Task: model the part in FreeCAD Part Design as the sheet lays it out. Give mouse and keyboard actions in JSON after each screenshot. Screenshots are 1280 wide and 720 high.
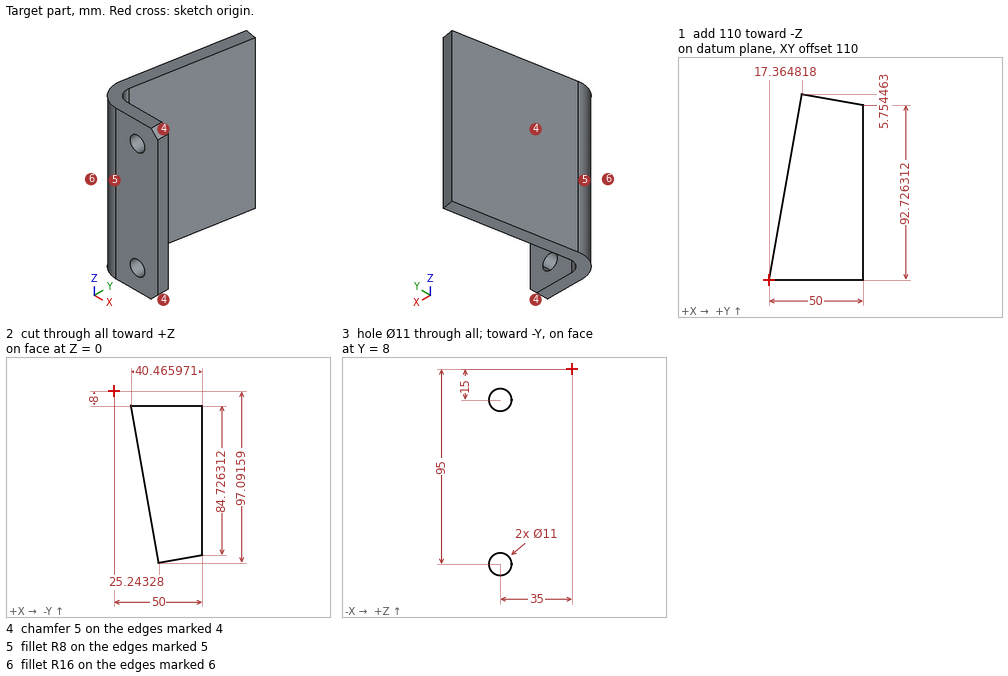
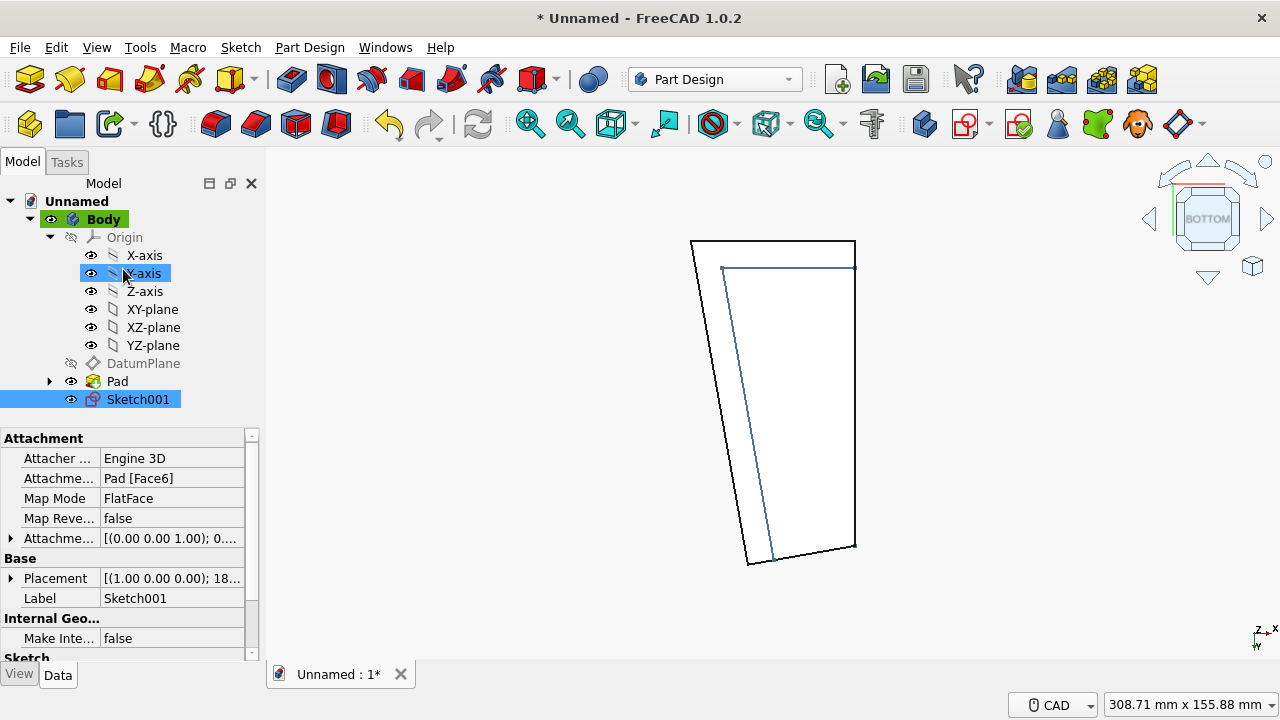
{"action": "left_click", "coordinate": [292, 80]}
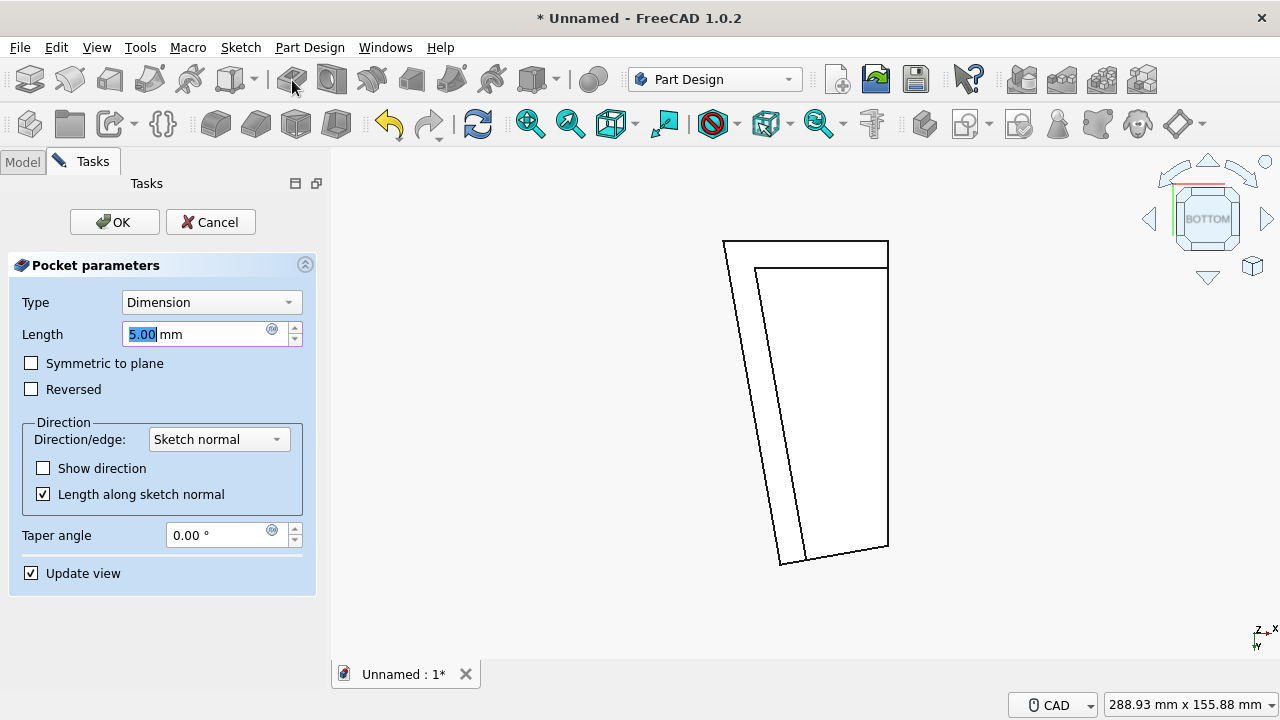
{"action": "left_click", "coordinate": [212, 302]}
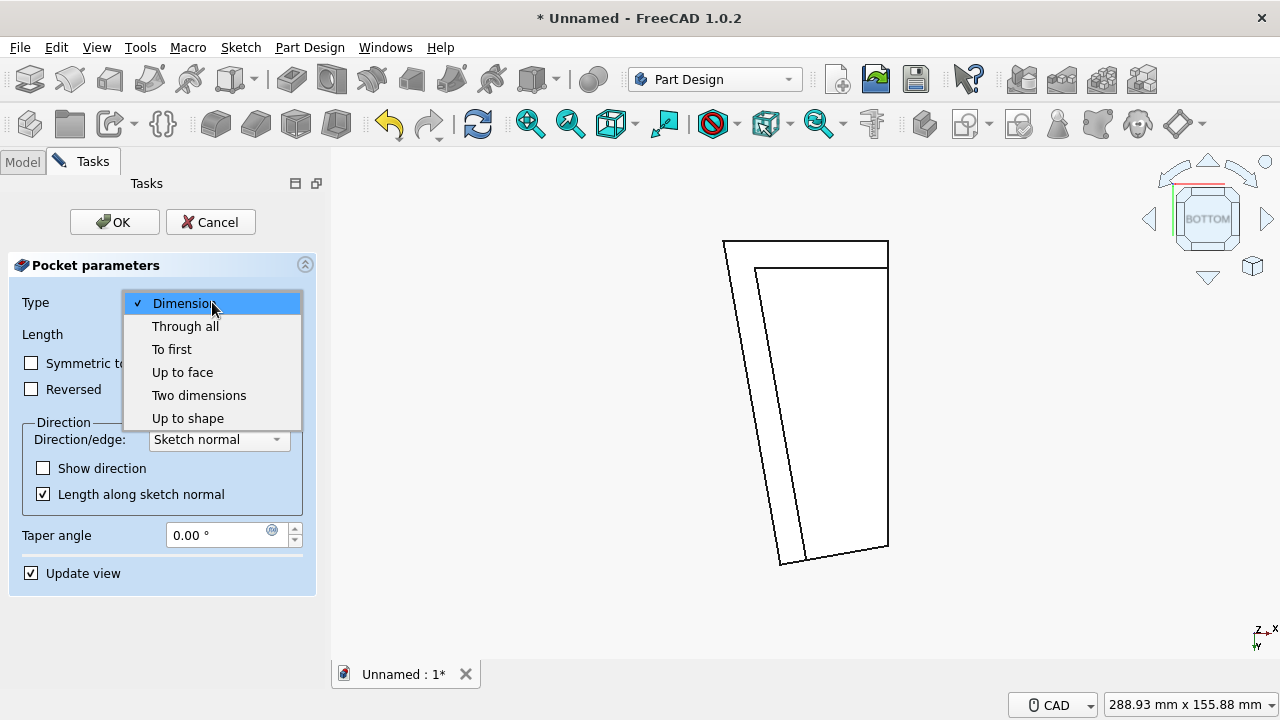
{"action": "left_click", "coordinate": [212, 326]}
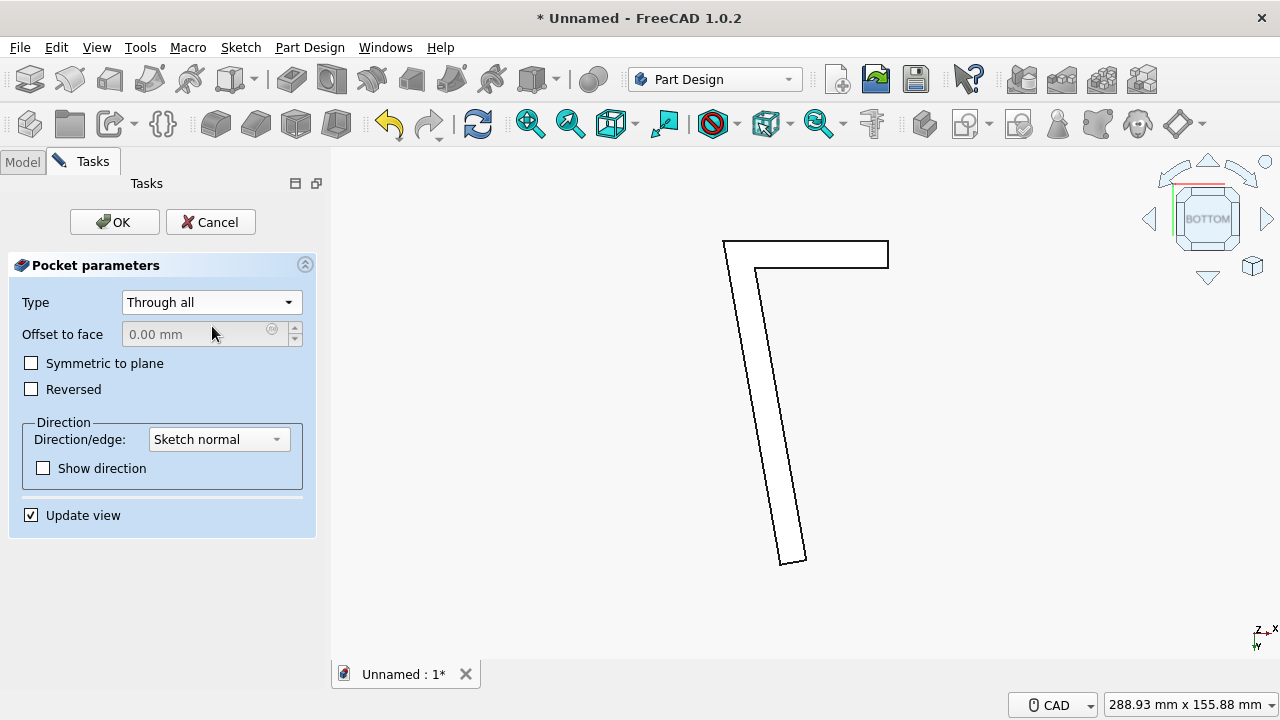
{"action": "left_click", "coordinate": [115, 222]}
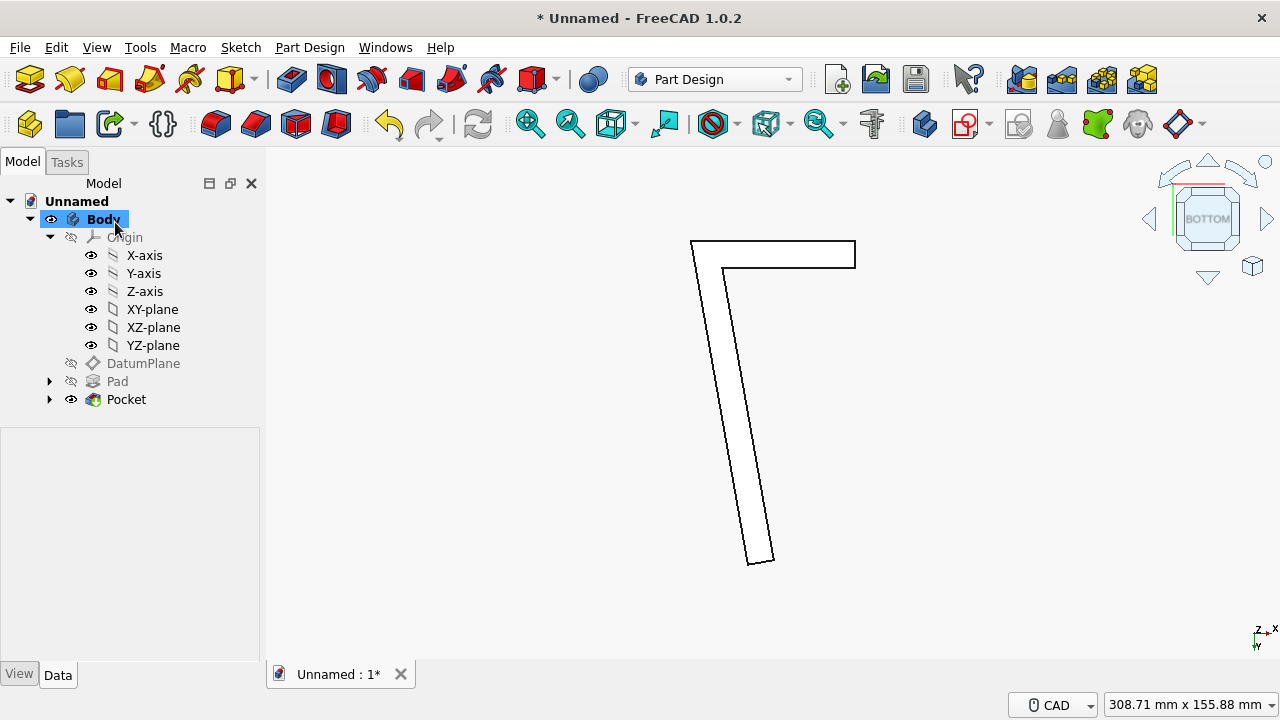
{"action": "key", "text": "4"}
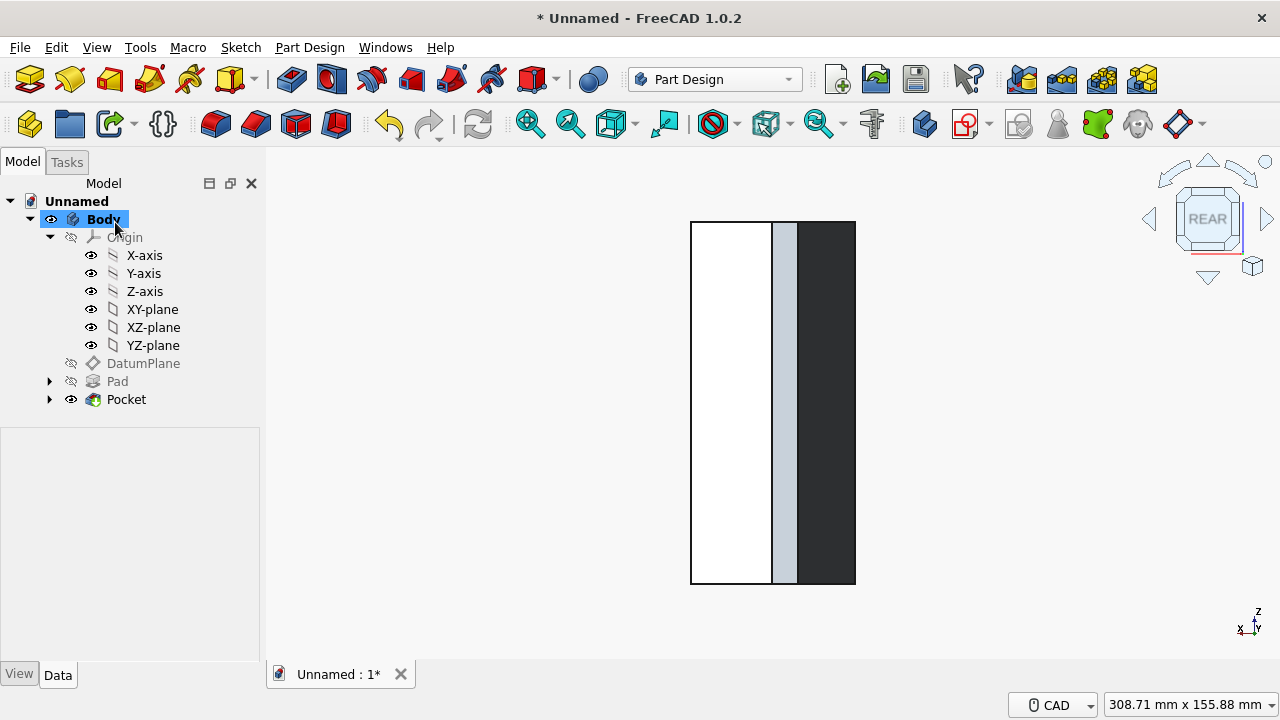
{"action": "left_click", "coordinate": [757, 299]}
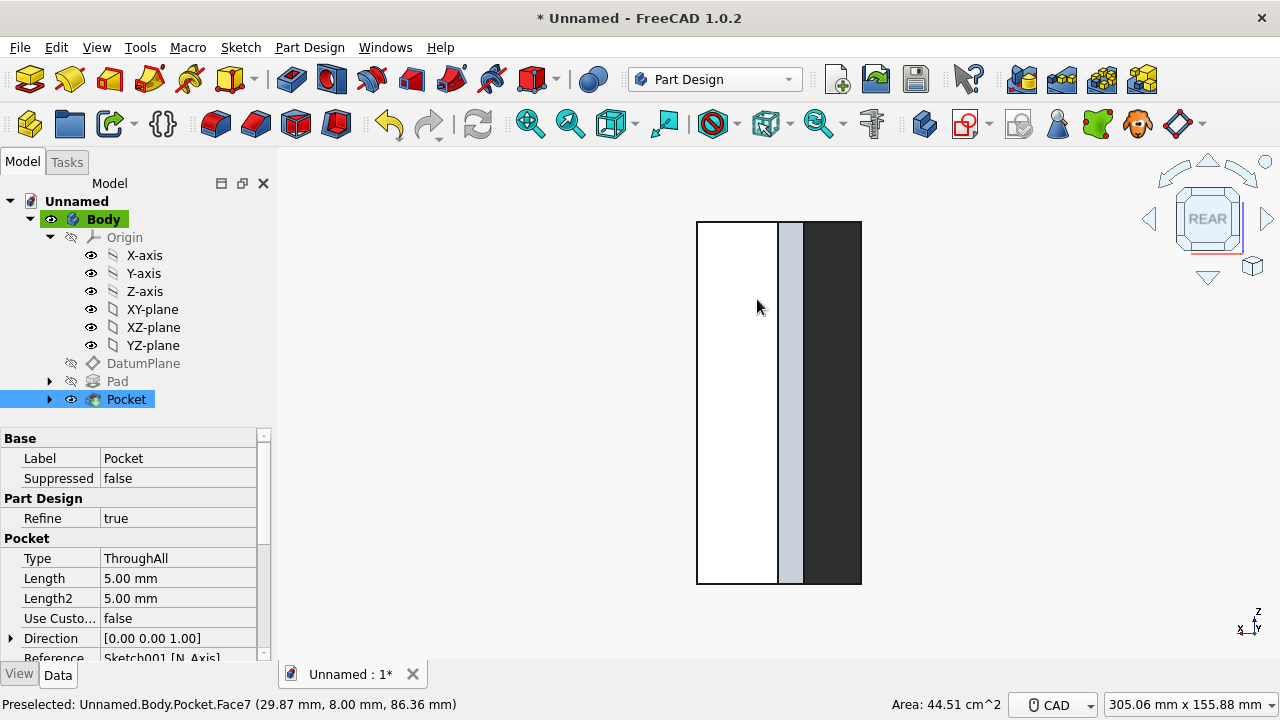
{"action": "left_click", "coordinate": [966, 124]}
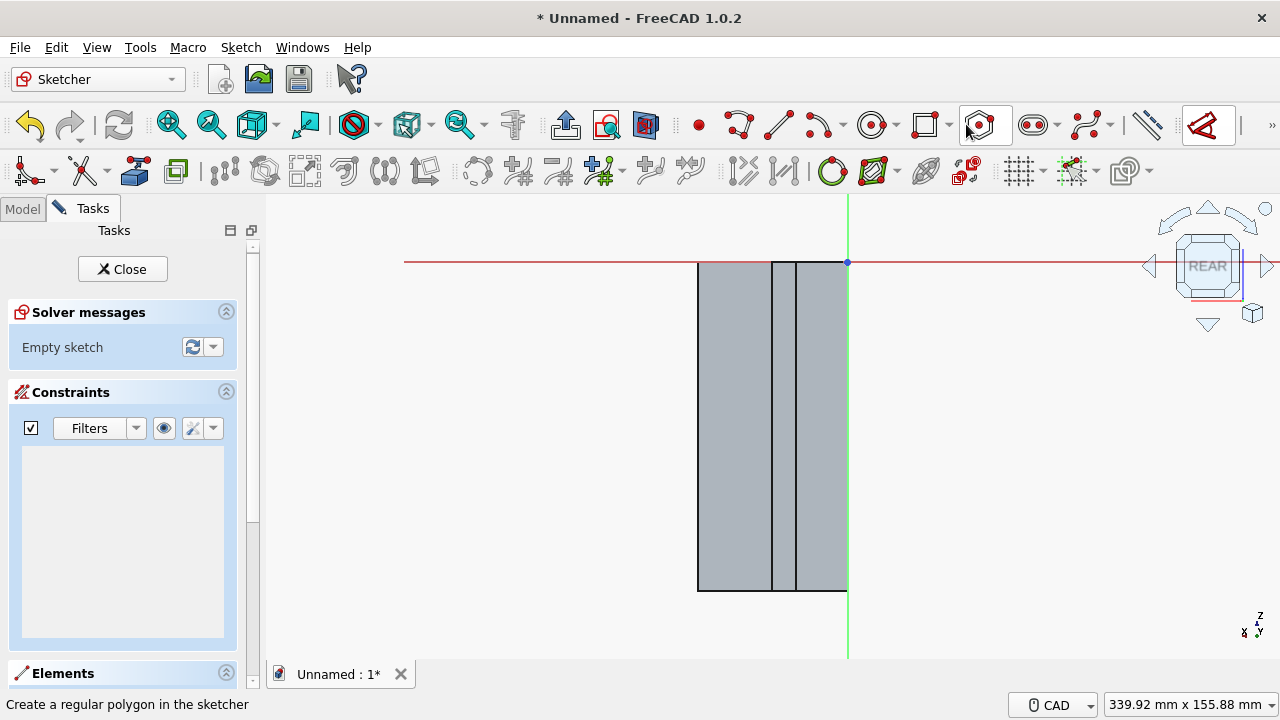
{"action": "left_click", "coordinate": [872, 126]}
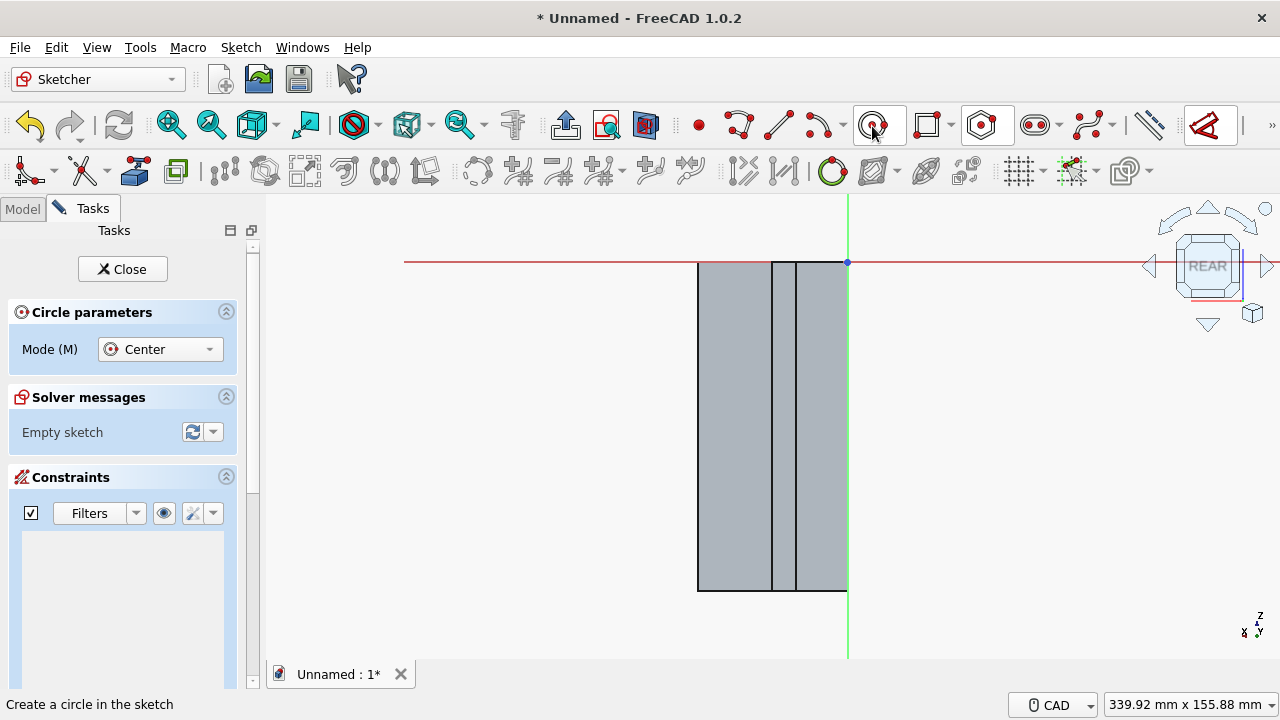
{"action": "scroll", "coordinate": [743, 546], "scroll_direction": "up", "scroll_amount": 2}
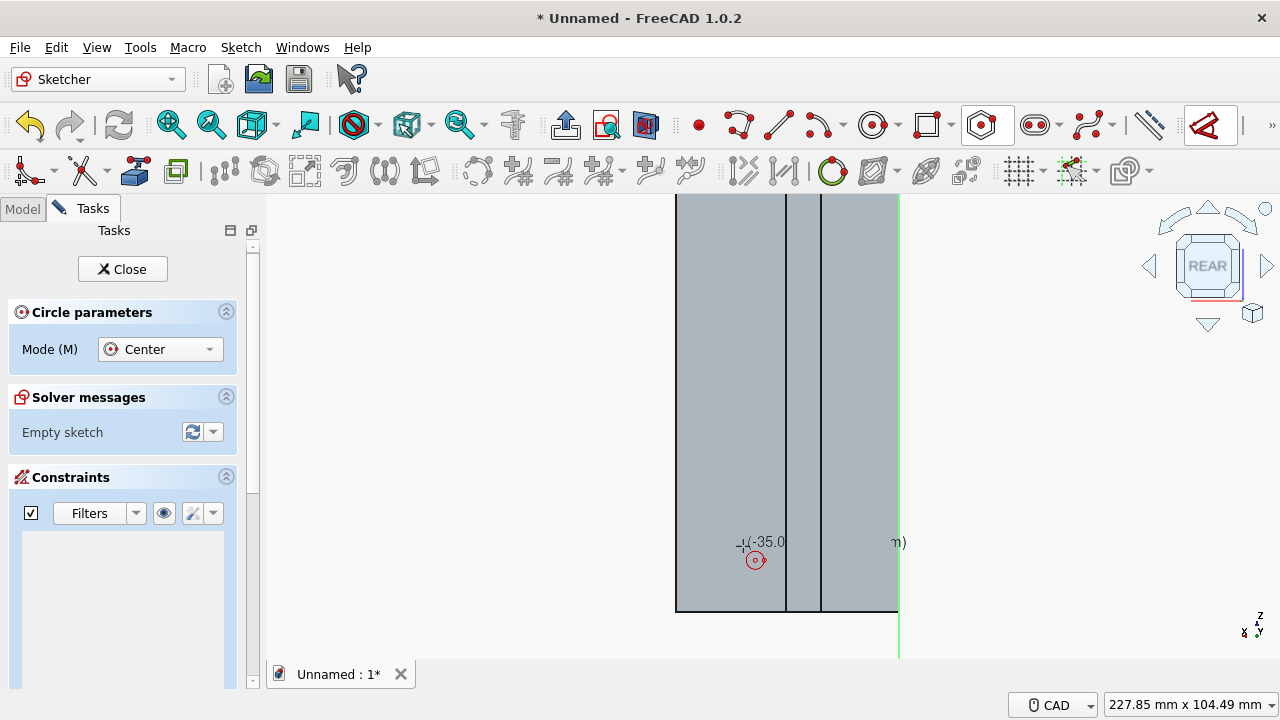
{"action": "left_click", "coordinate": [743, 545]}
{"action": "mouse_move", "coordinate": [760, 528]}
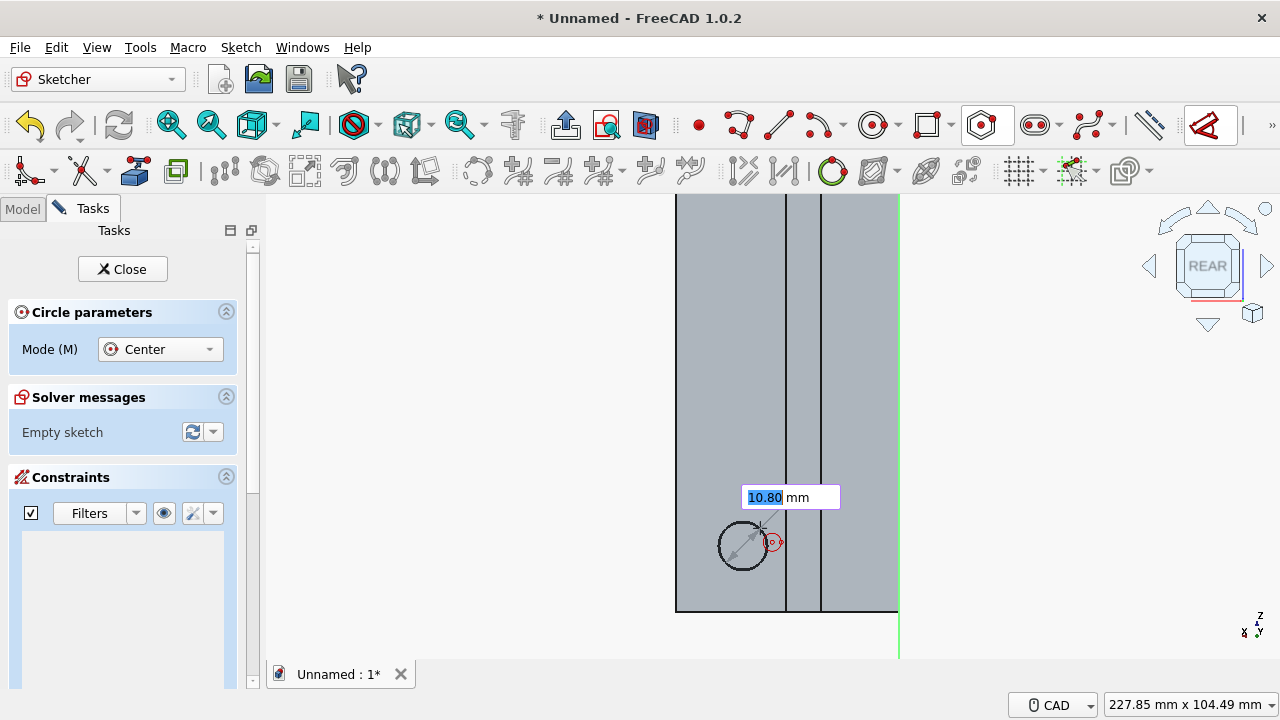
{"action": "type", "text": "11"}
{"action": "key", "text": "Return"}